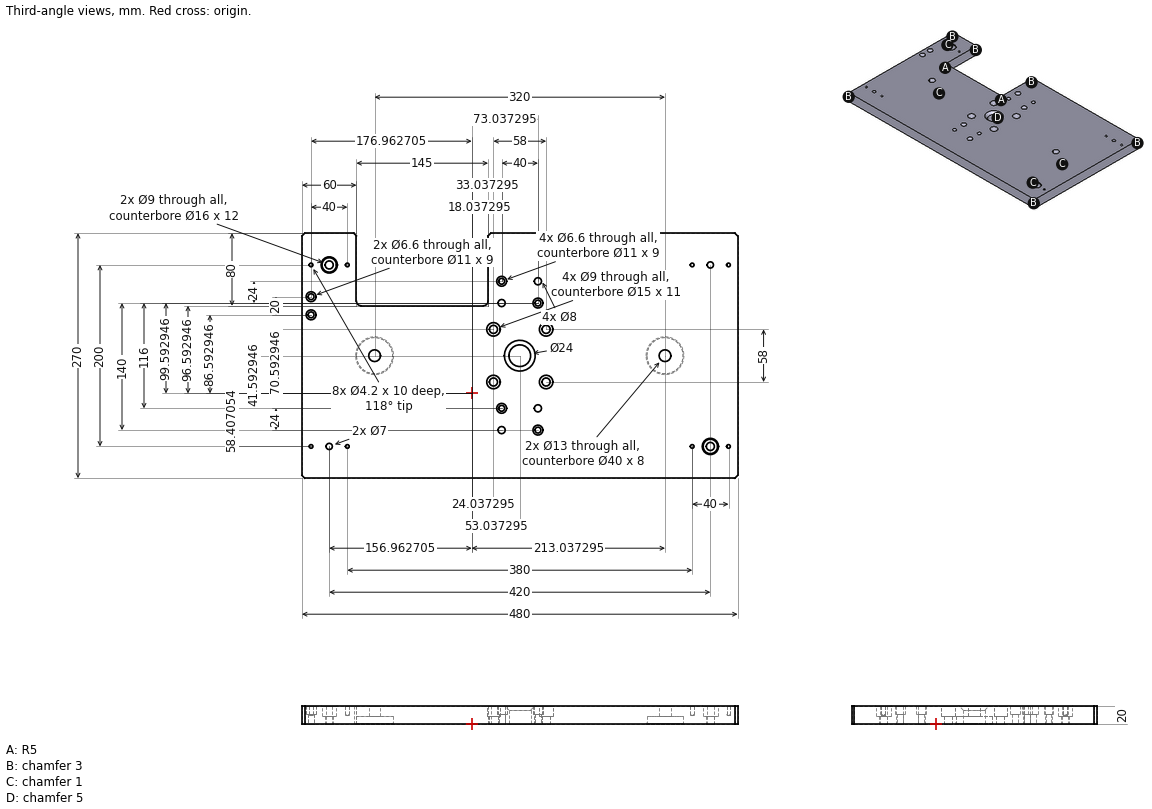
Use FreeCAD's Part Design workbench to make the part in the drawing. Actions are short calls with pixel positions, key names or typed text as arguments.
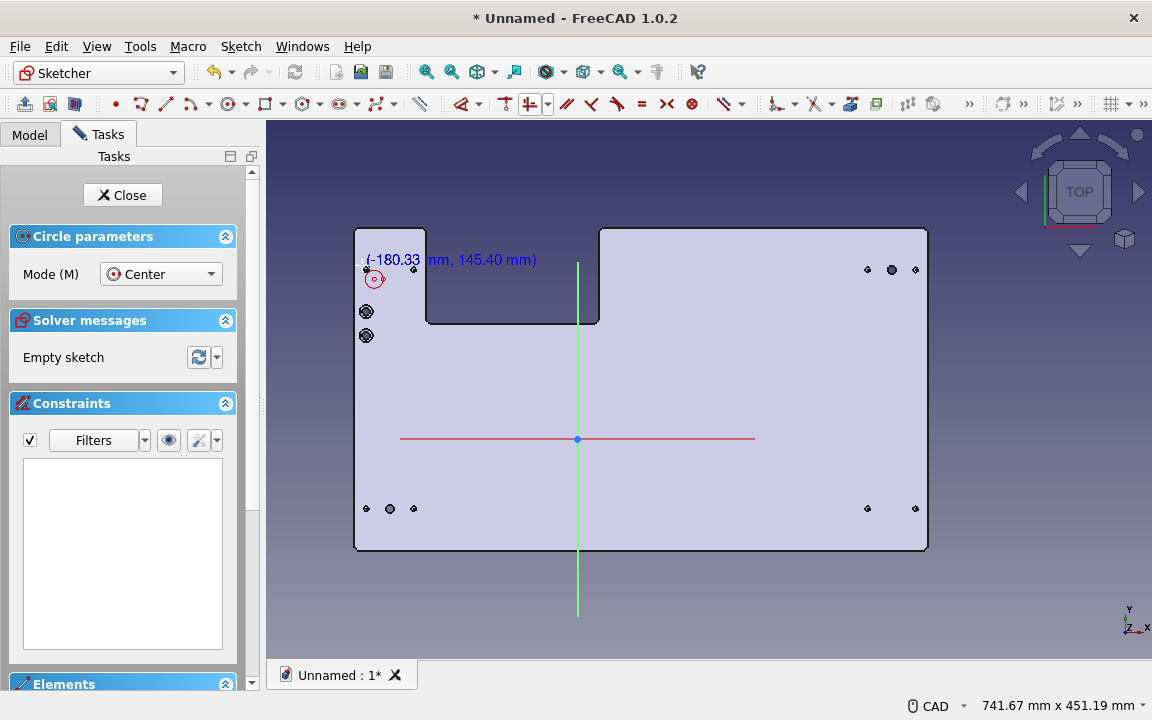
click(390, 270)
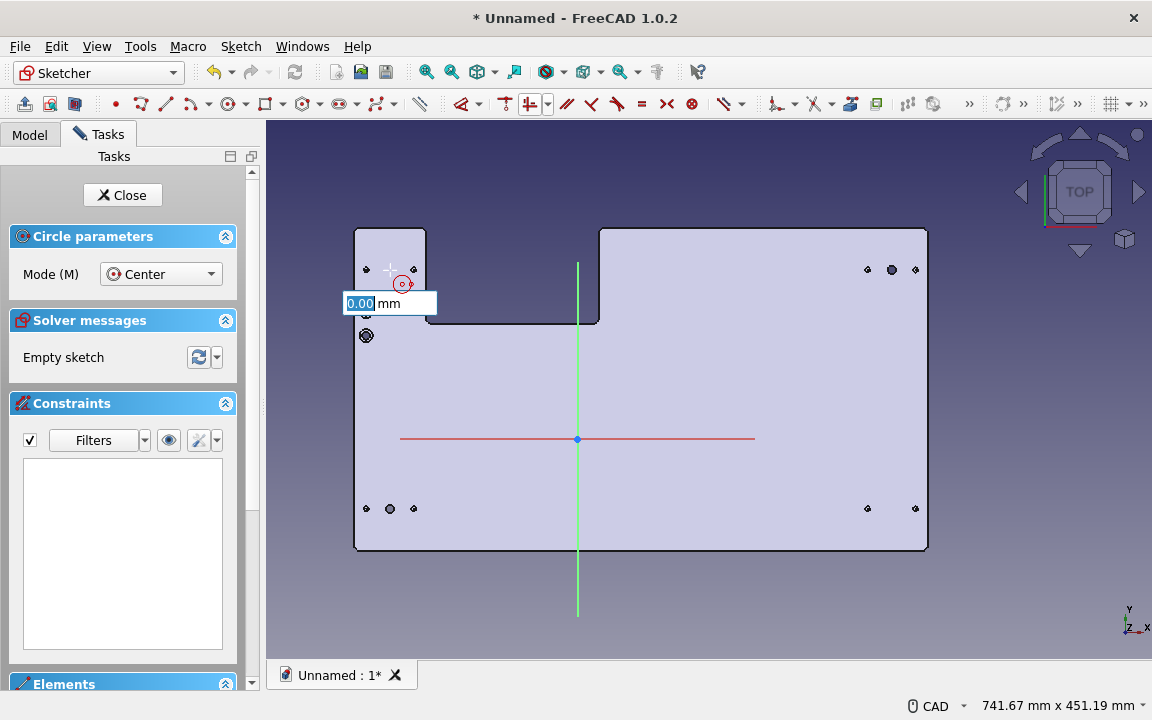
scroll(394, 266, up, 6)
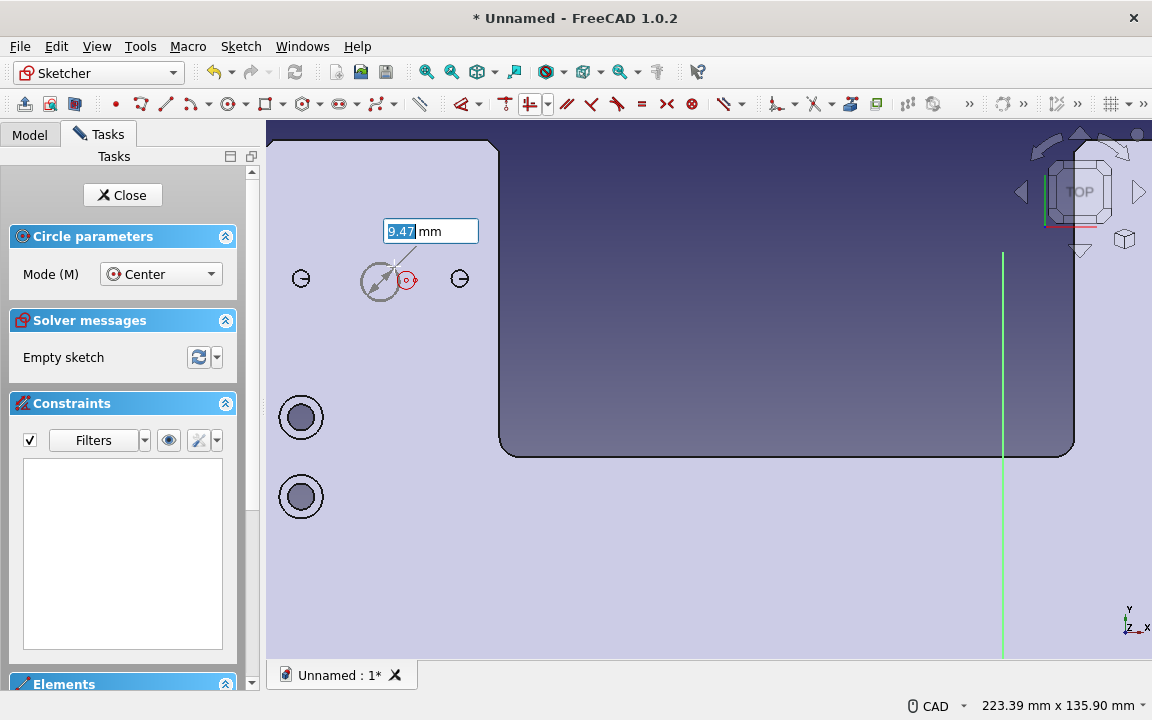
click(393, 266)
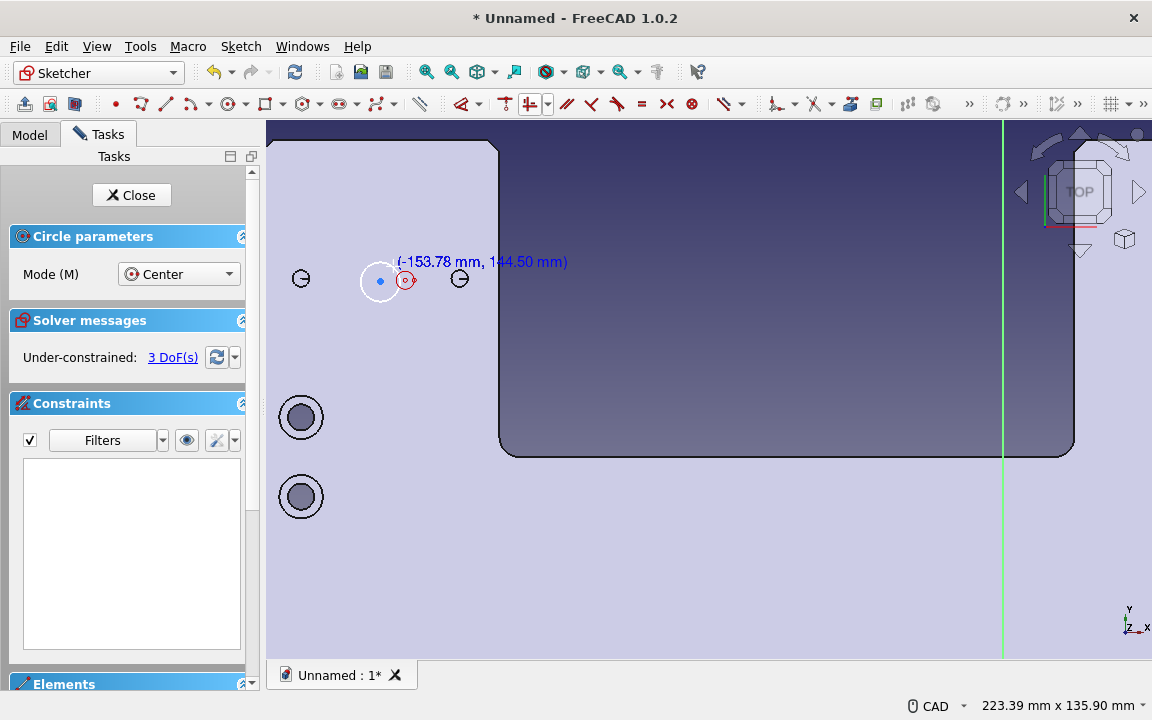
scroll(394, 266, down, 6)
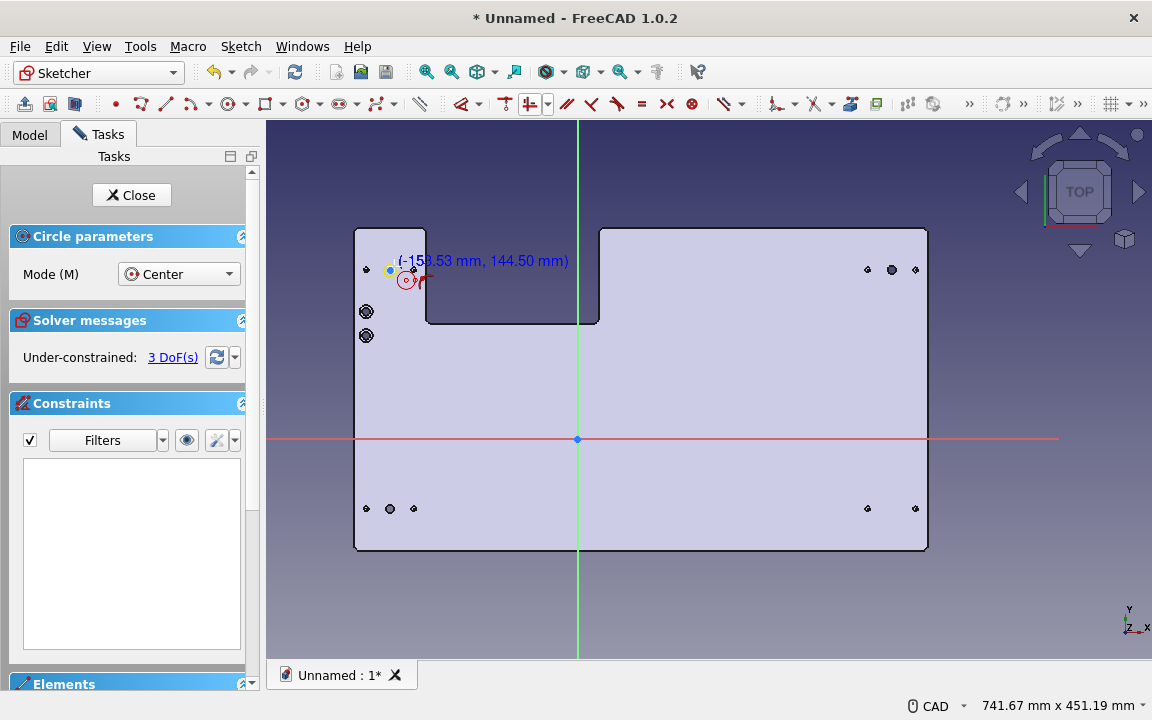
scroll(892, 509, up, 8)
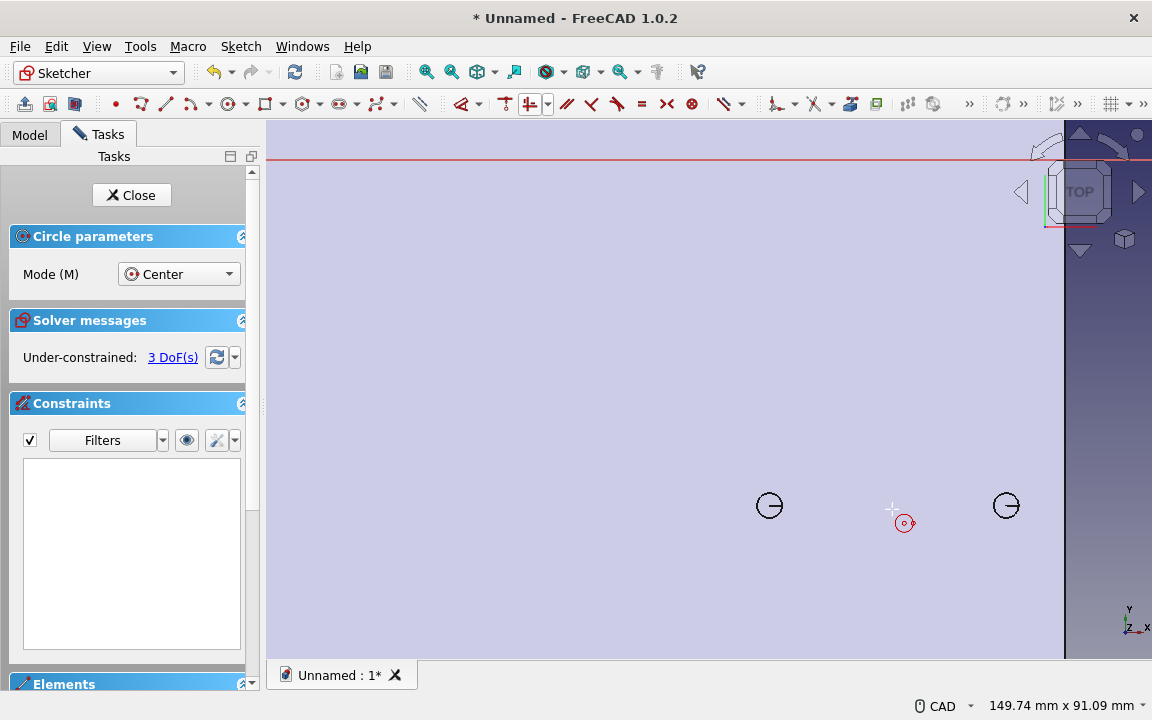
scroll(892, 510, down, 8)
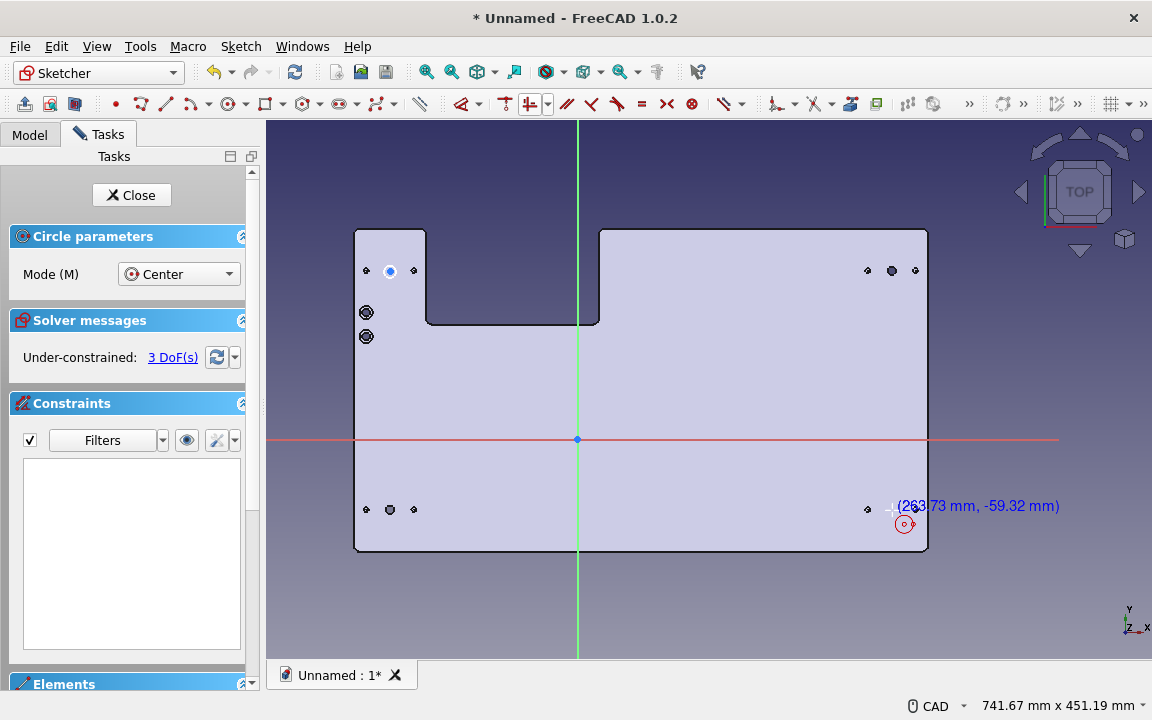
click(892, 510)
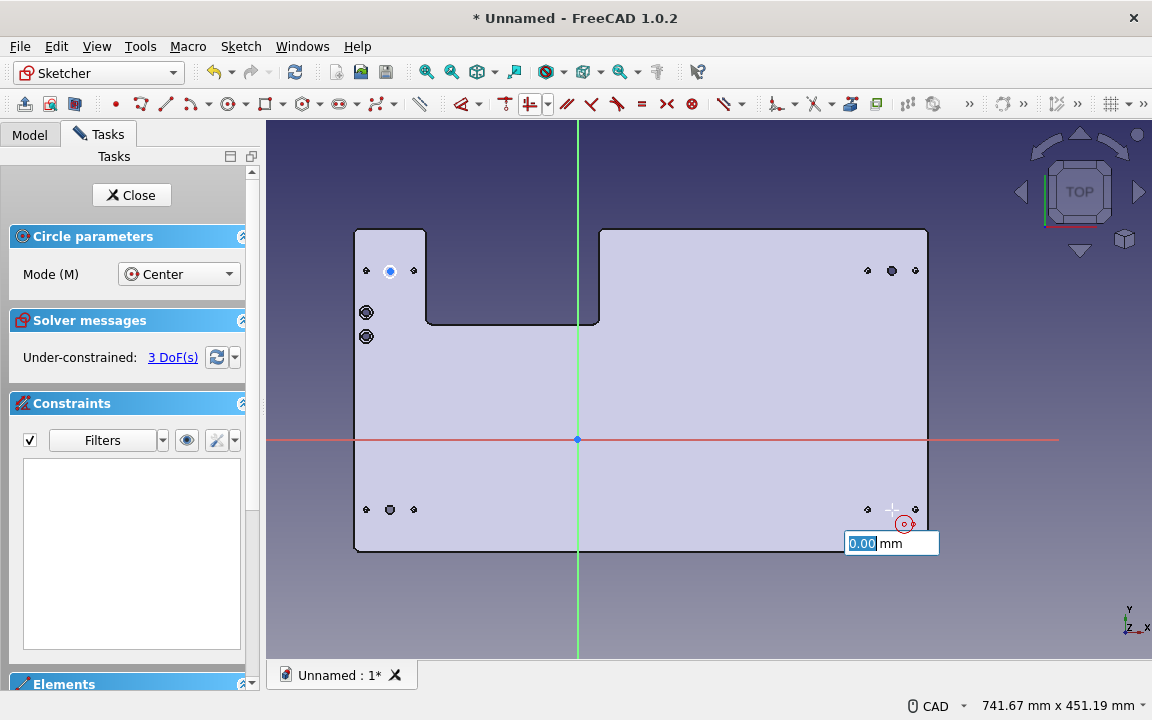
scroll(896, 506, up, 6)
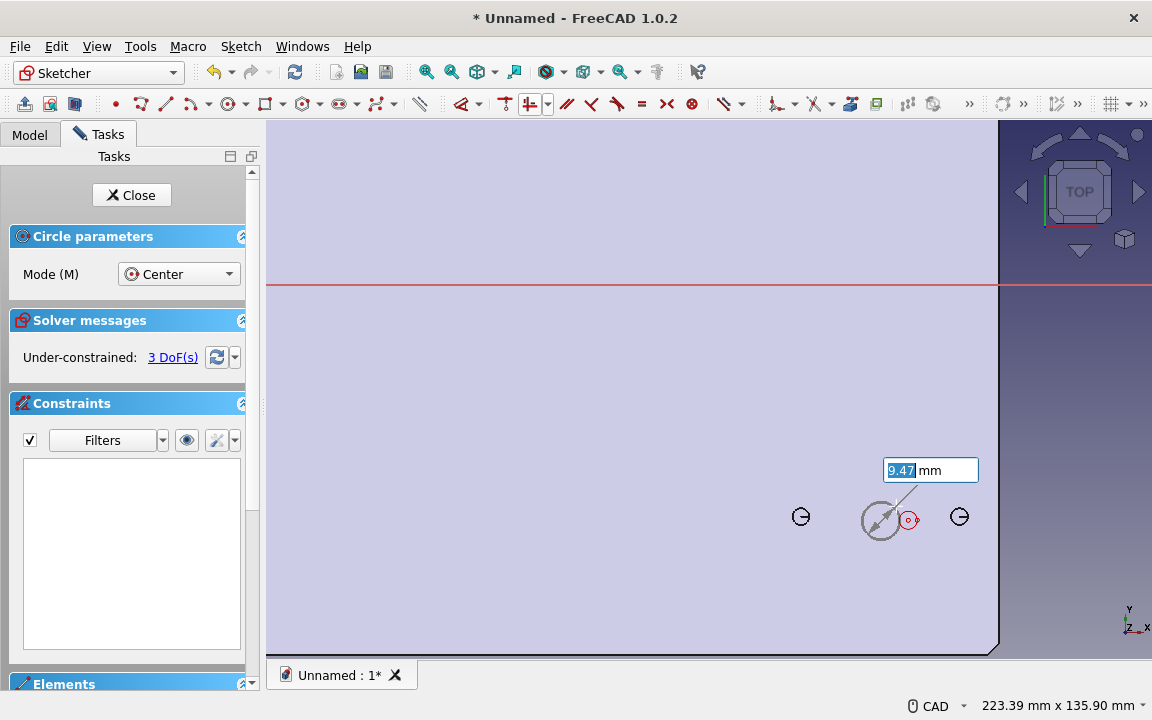
click(893, 504)
key(Escape)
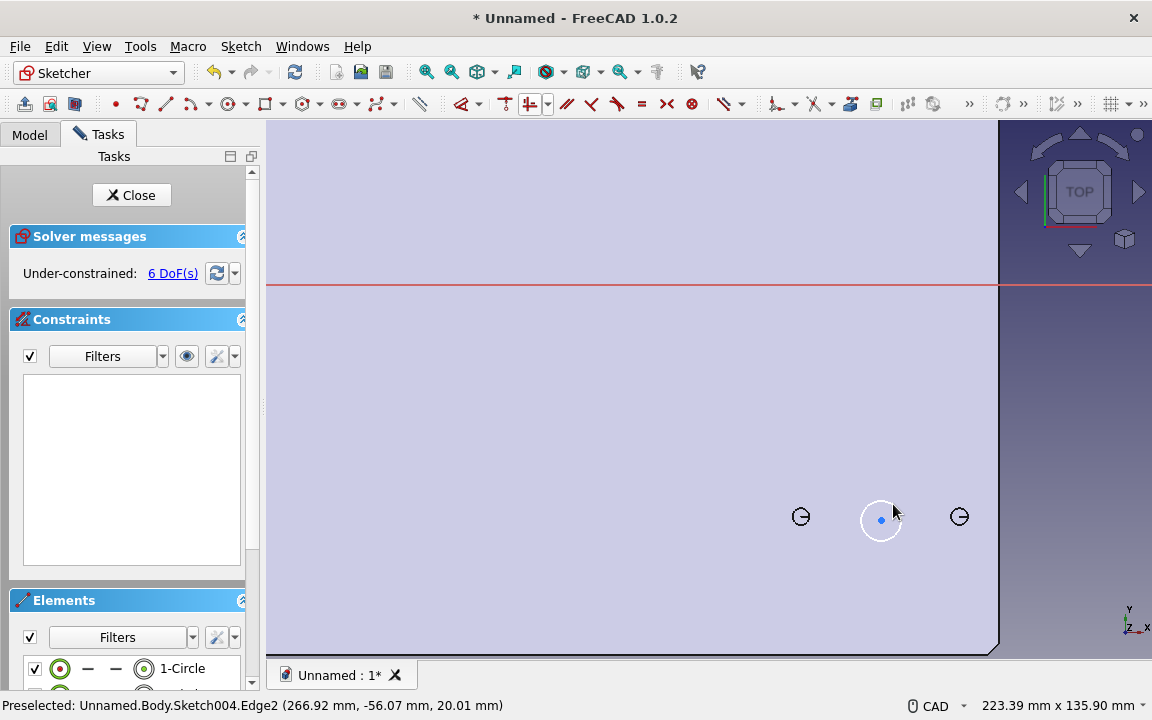
scroll(896, 506, down, 6)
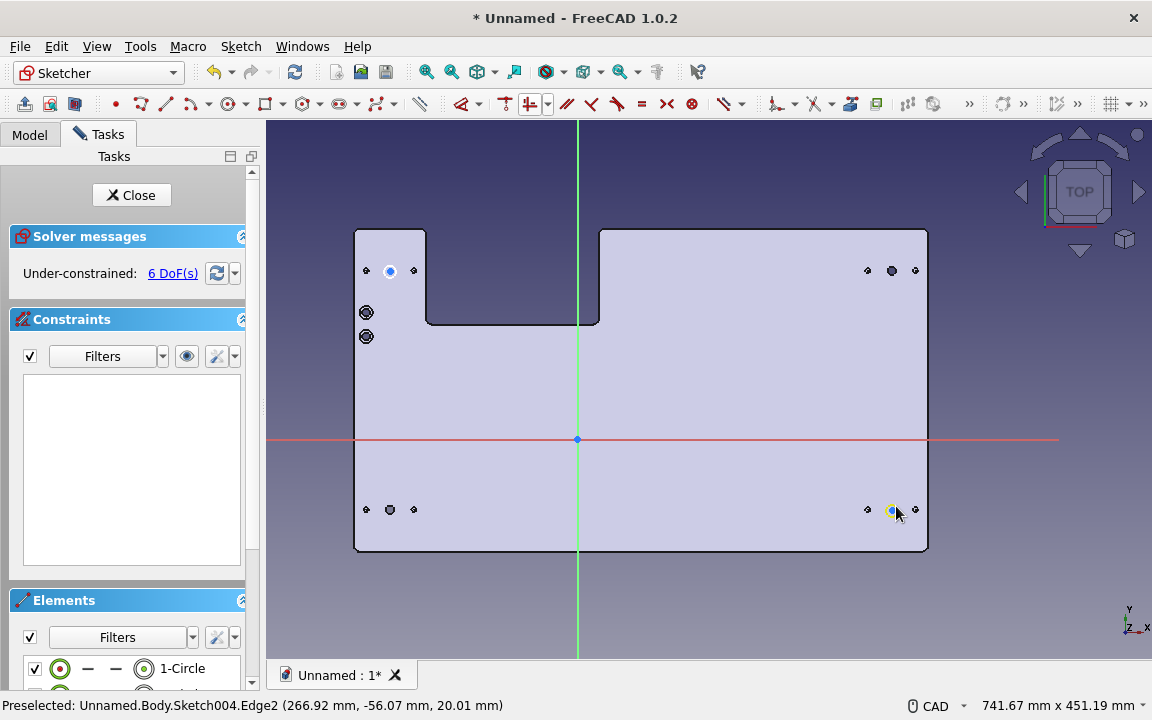
scroll(394, 268, up, 5)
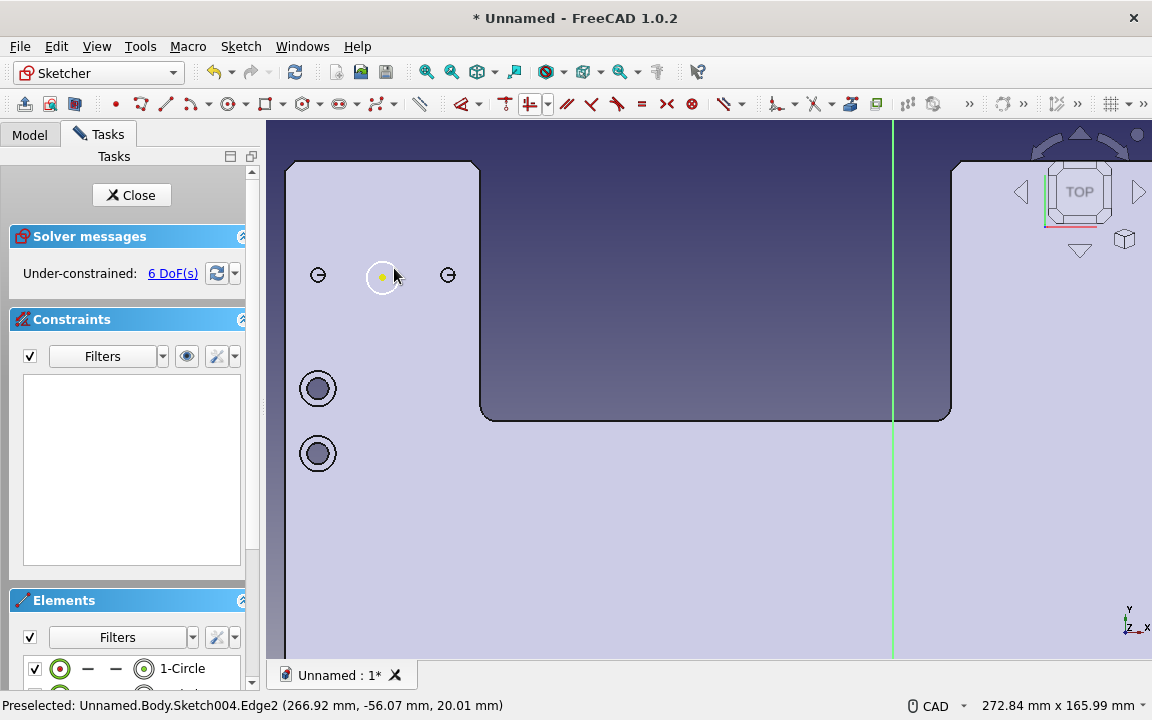
click(394, 266)